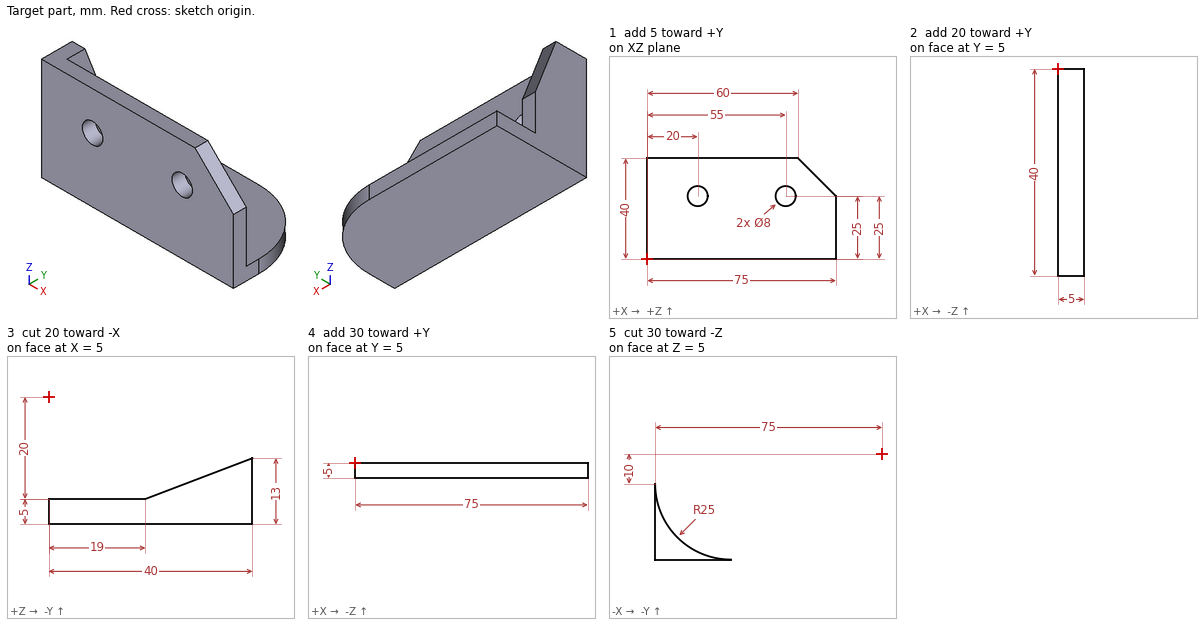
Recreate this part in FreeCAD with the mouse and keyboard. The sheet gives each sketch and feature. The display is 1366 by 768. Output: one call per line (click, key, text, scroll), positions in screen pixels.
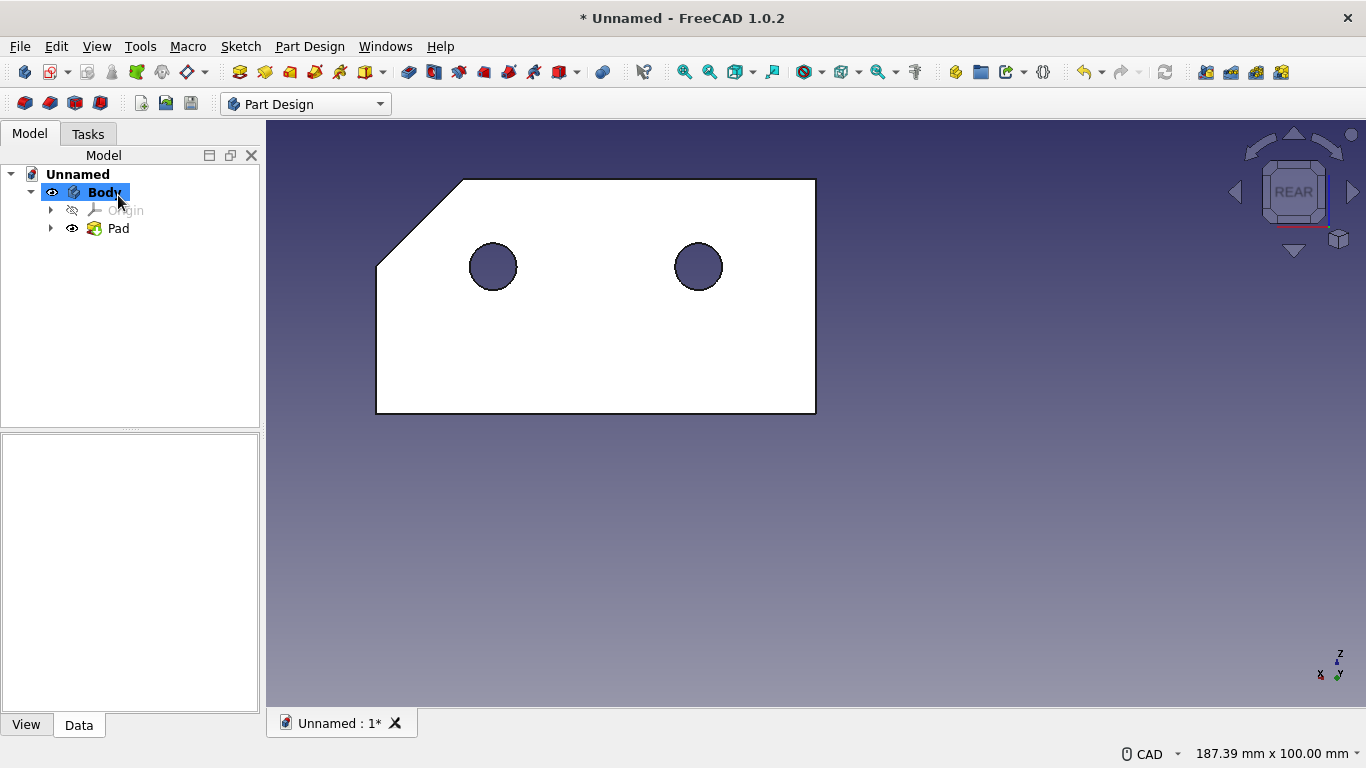
click(685, 72)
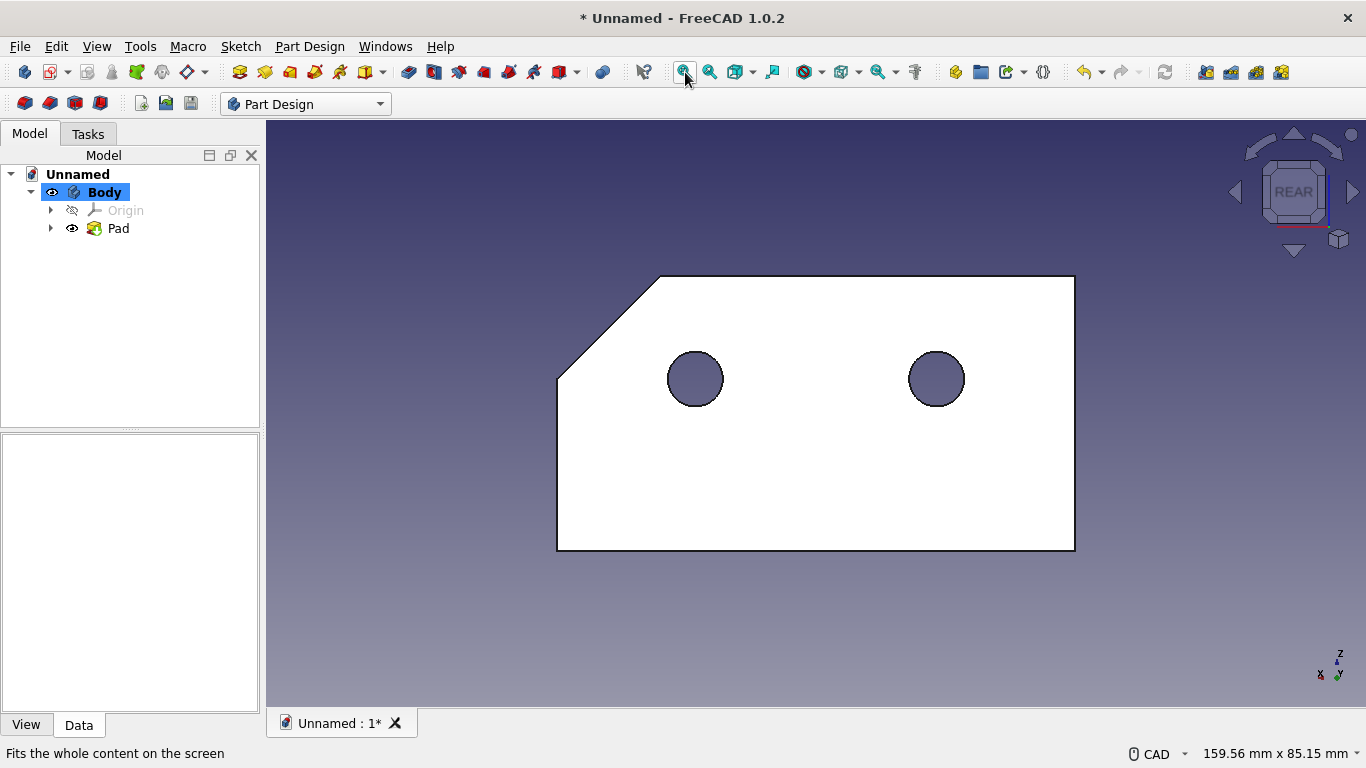
click(816, 452)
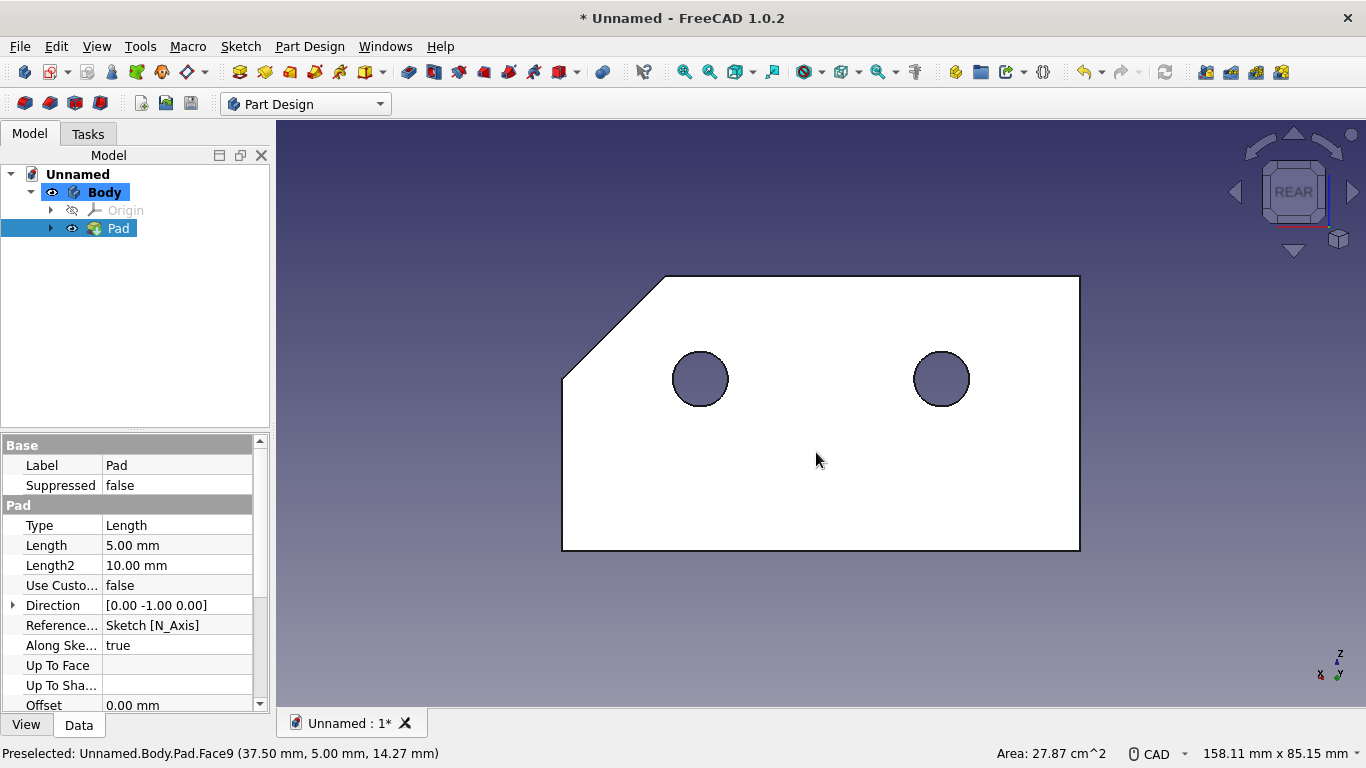
click(50, 72)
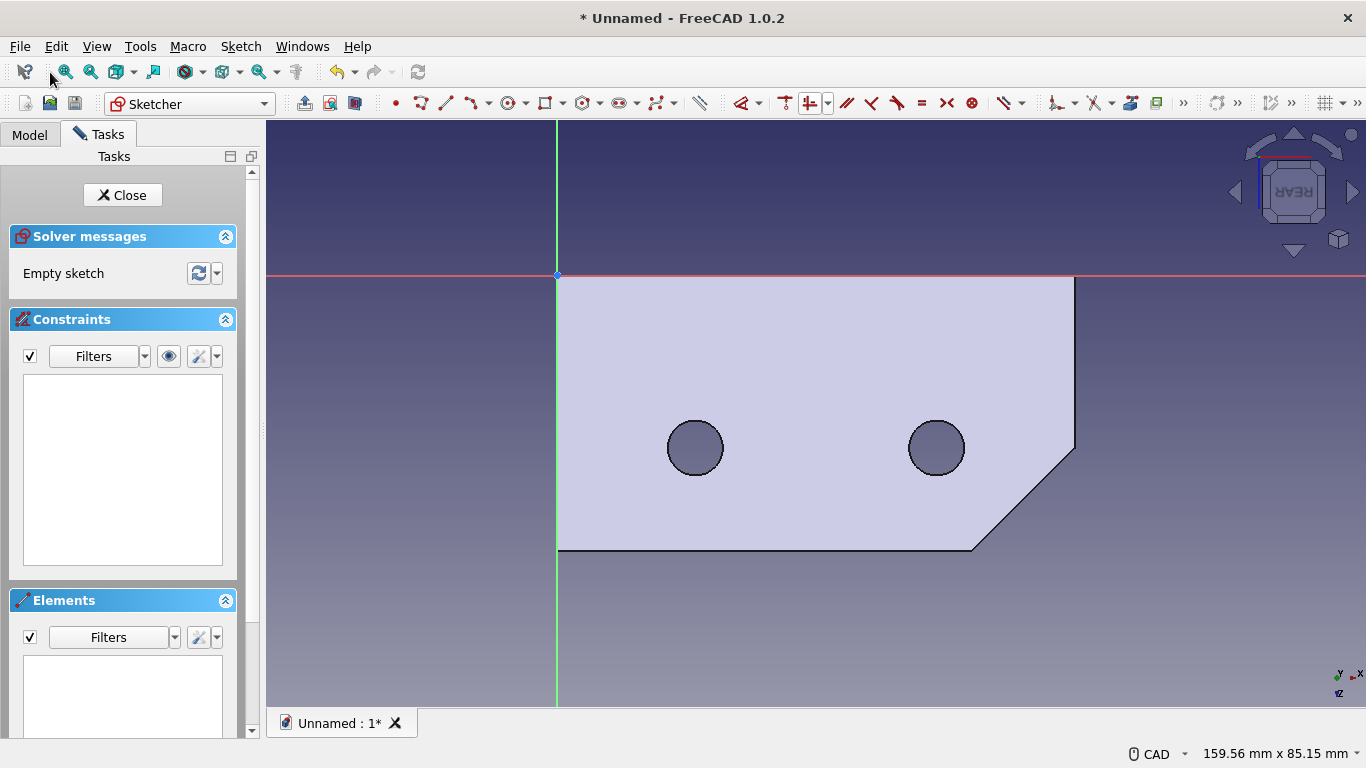
scroll(294, 413, up, 2)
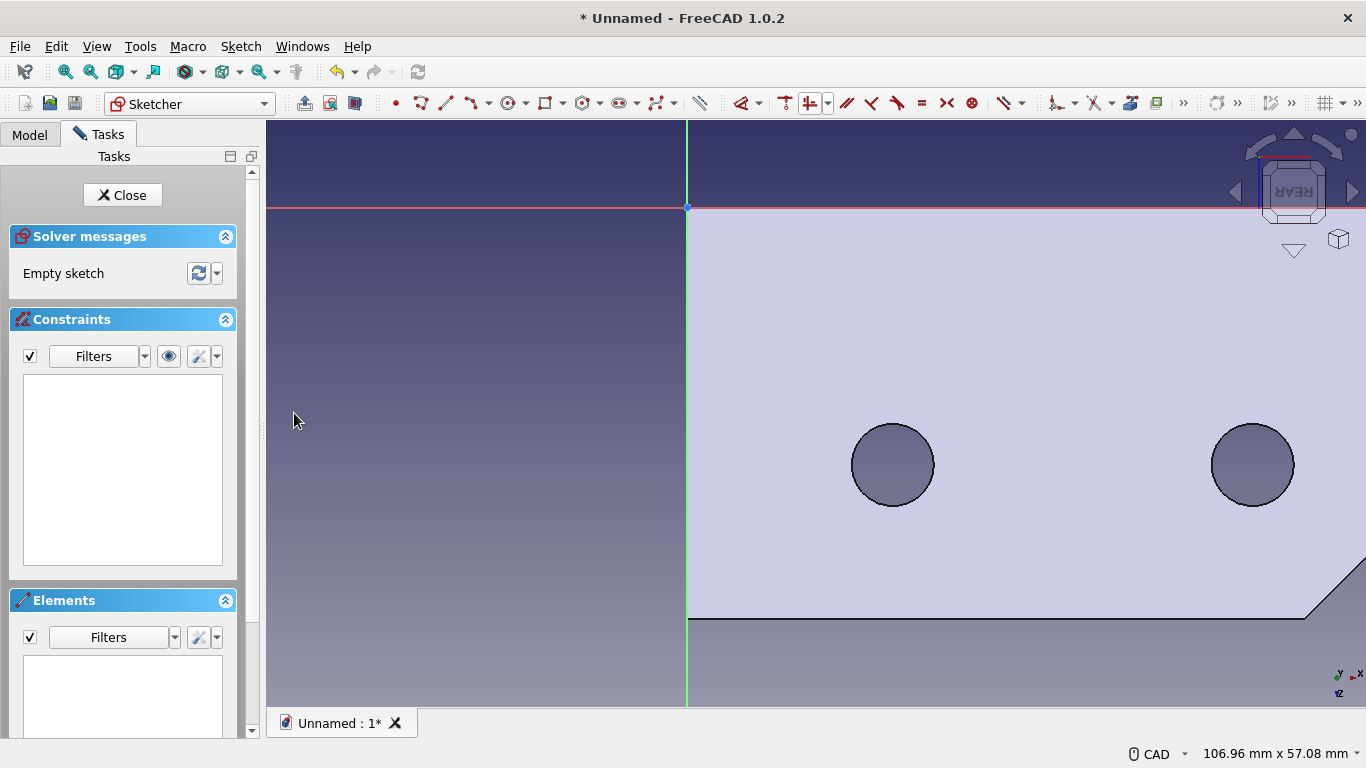
click(544, 104)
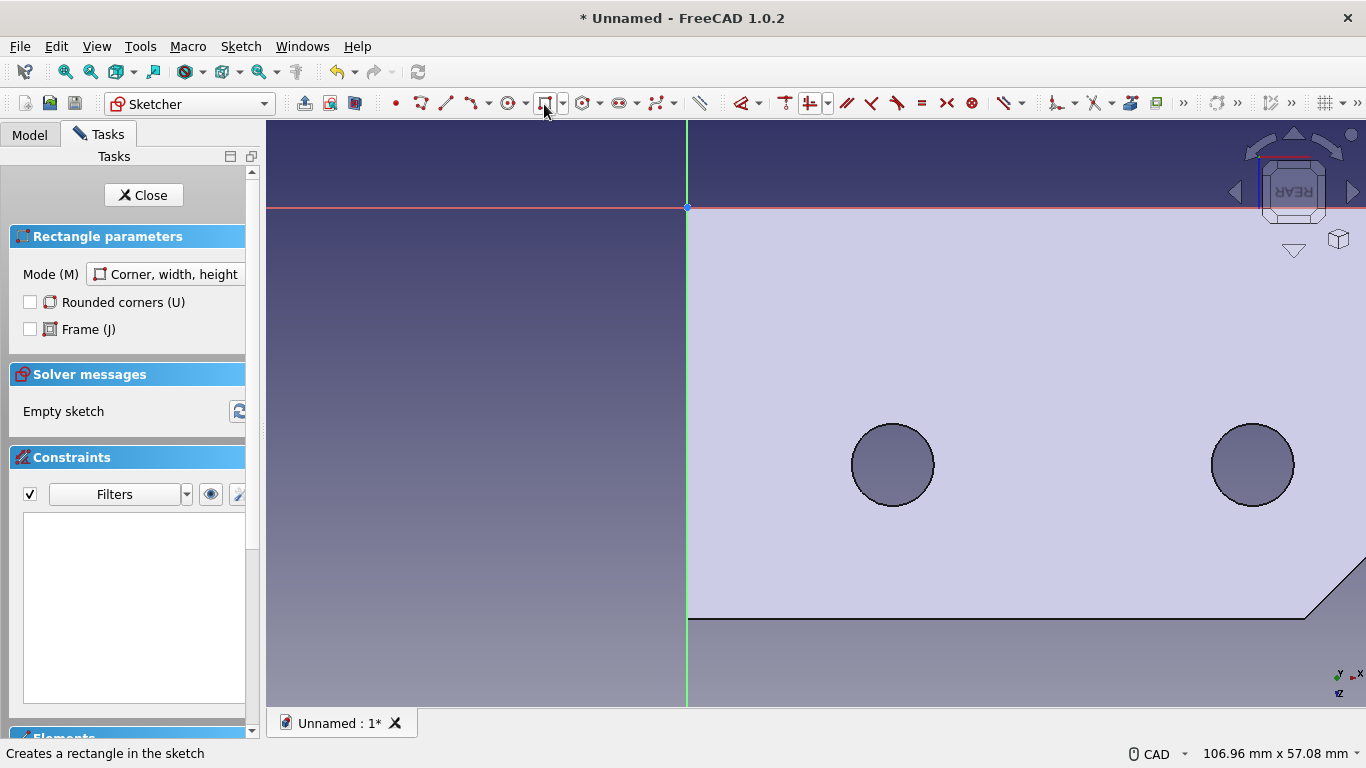
click(687, 208)
click(738, 619)
key(Escape)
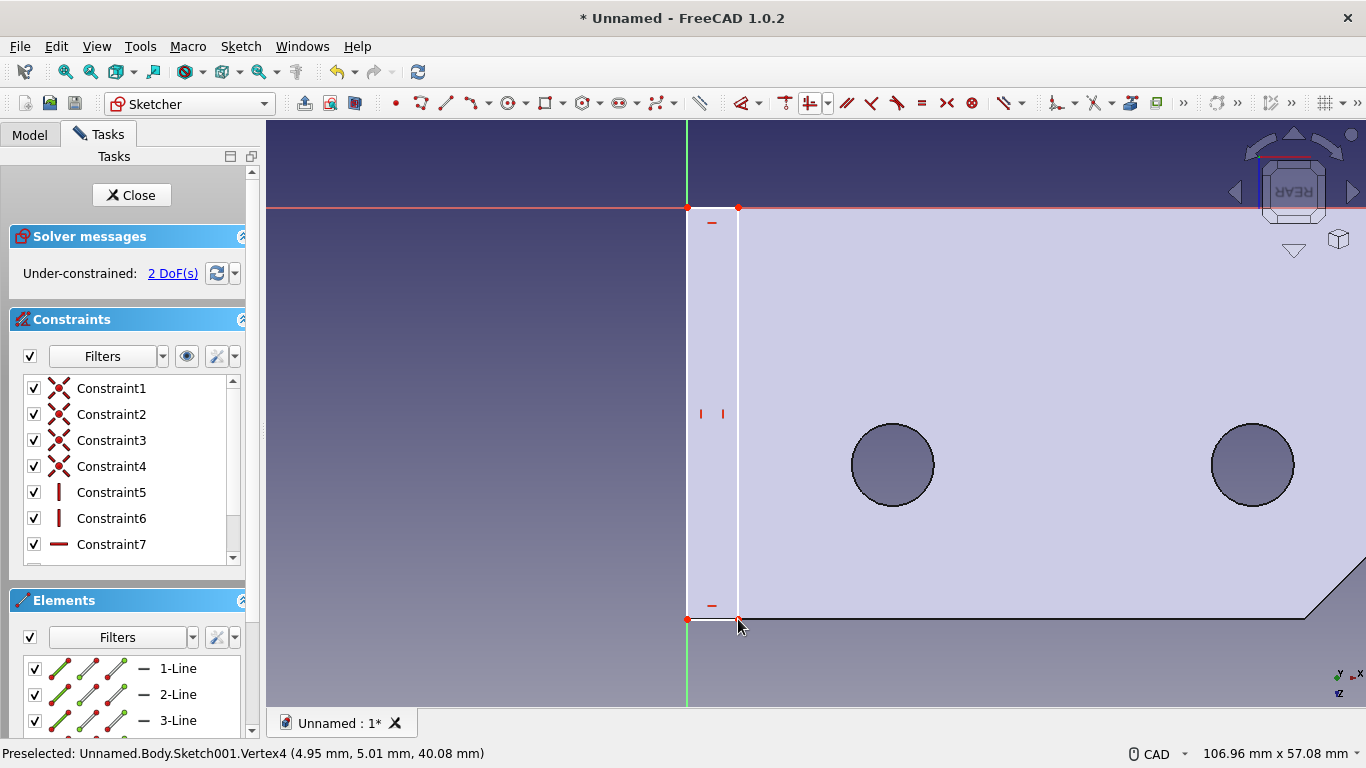
click(740, 104)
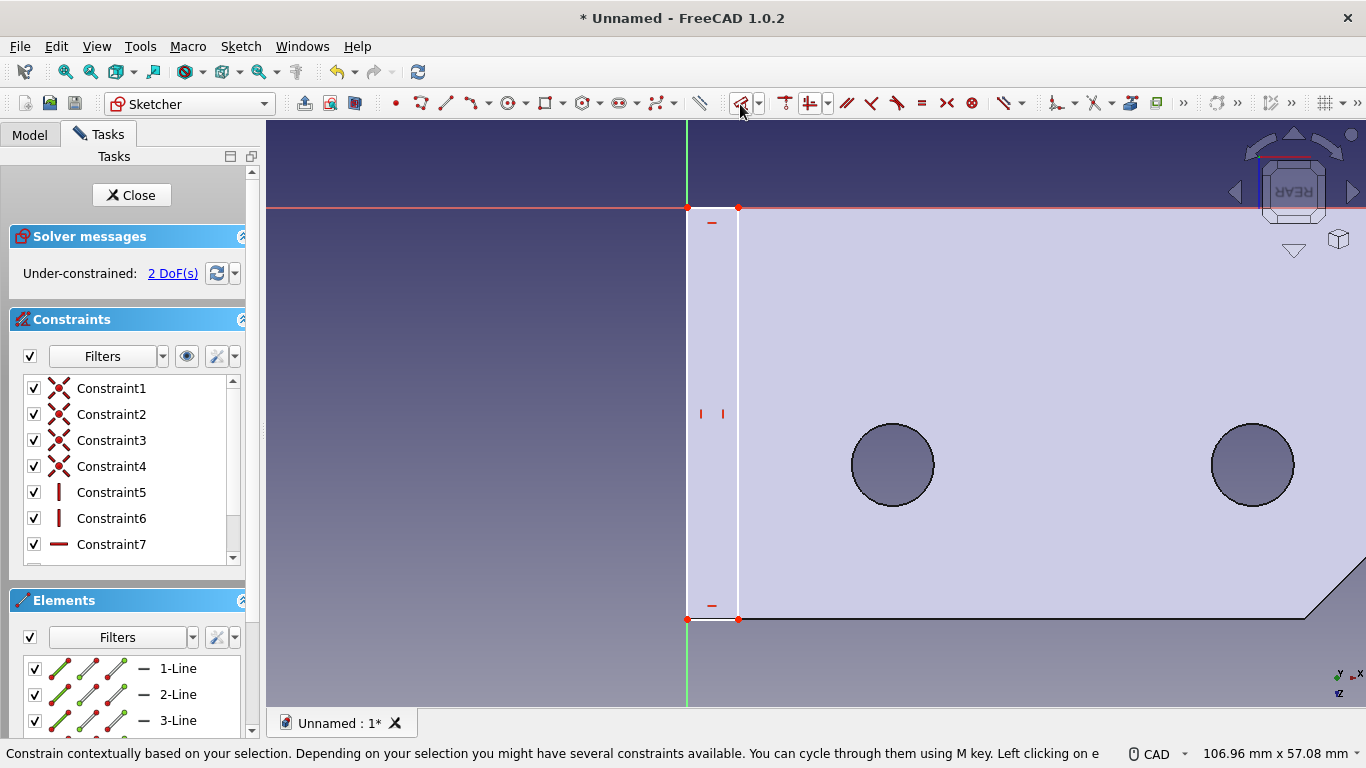
click(702, 620)
click(713, 654)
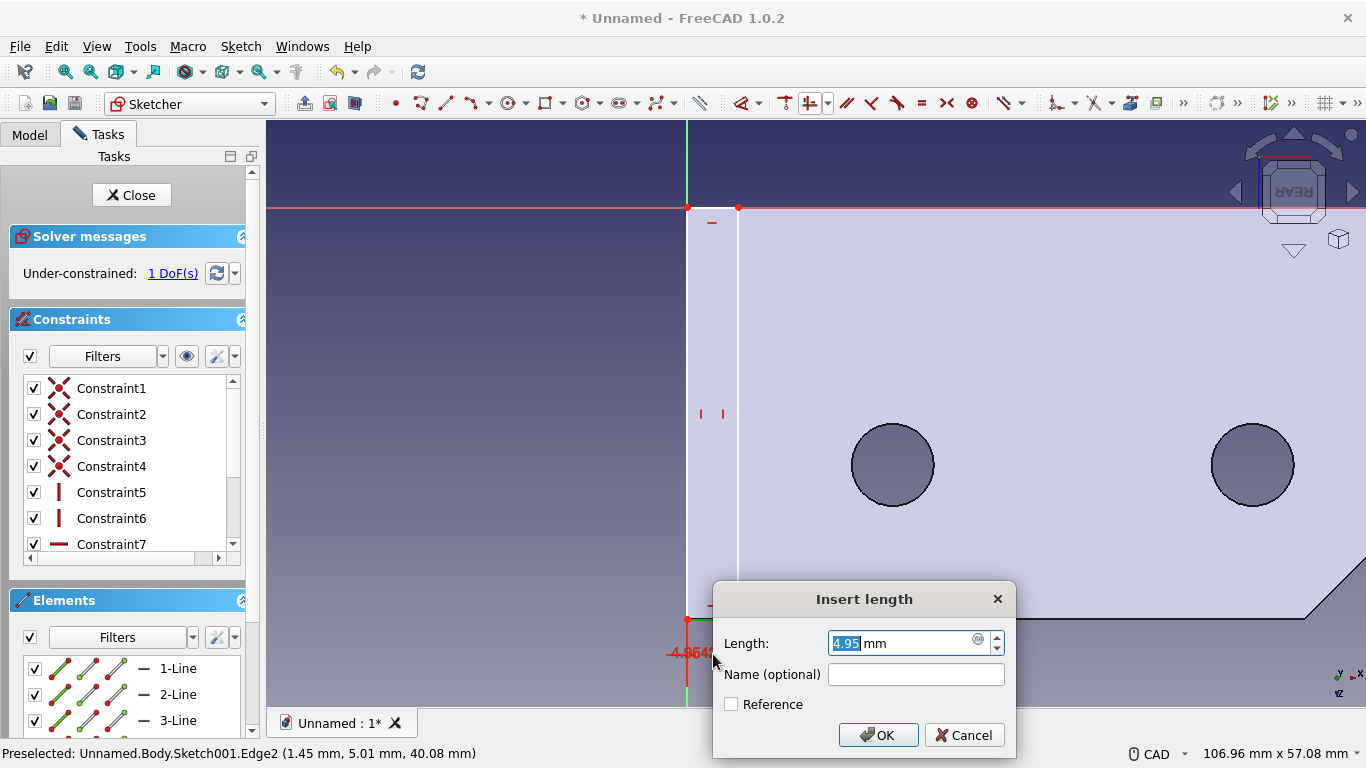
text(5)
key(Return)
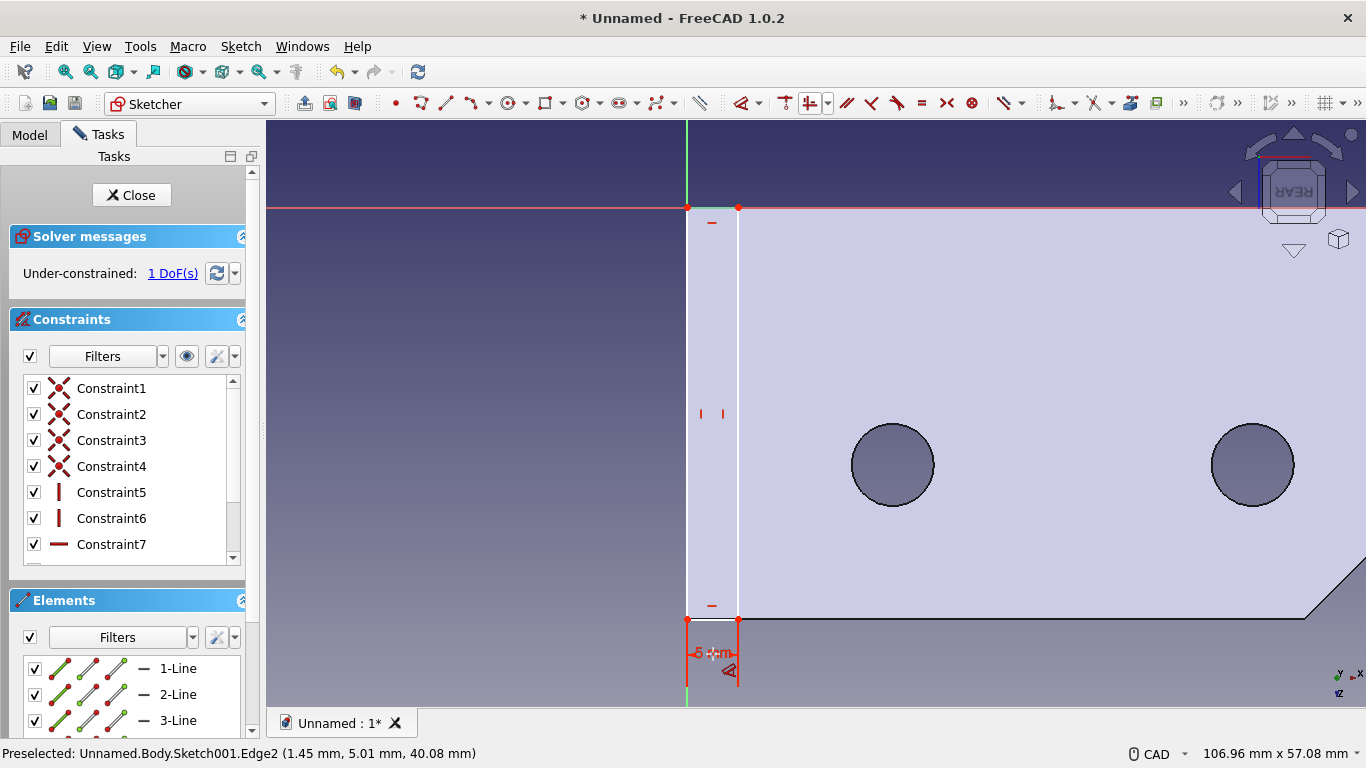
click(687, 331)
click(653, 414)